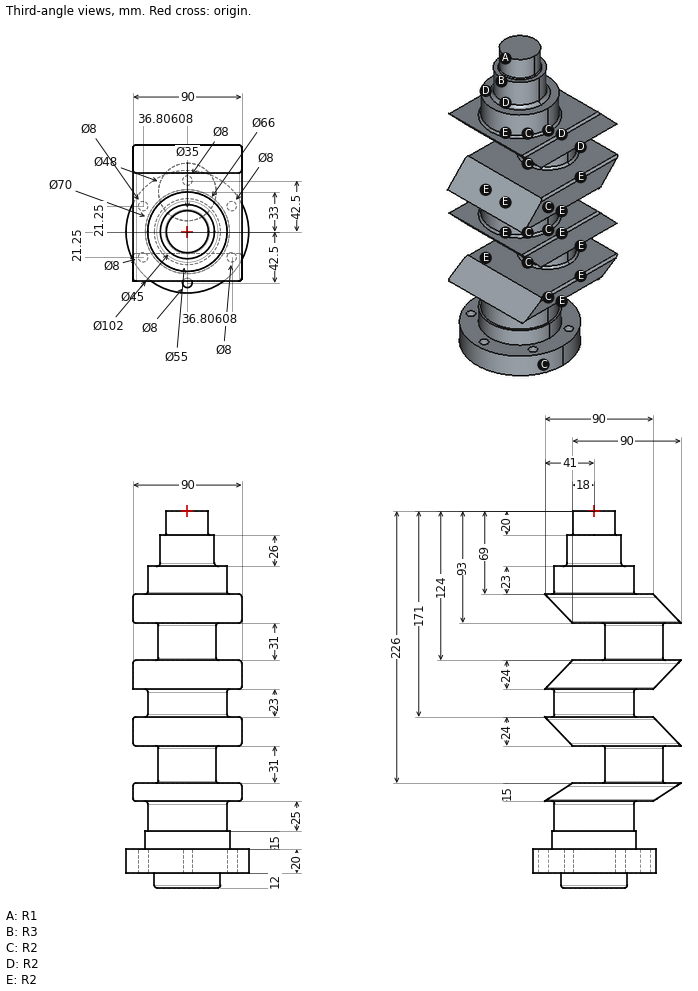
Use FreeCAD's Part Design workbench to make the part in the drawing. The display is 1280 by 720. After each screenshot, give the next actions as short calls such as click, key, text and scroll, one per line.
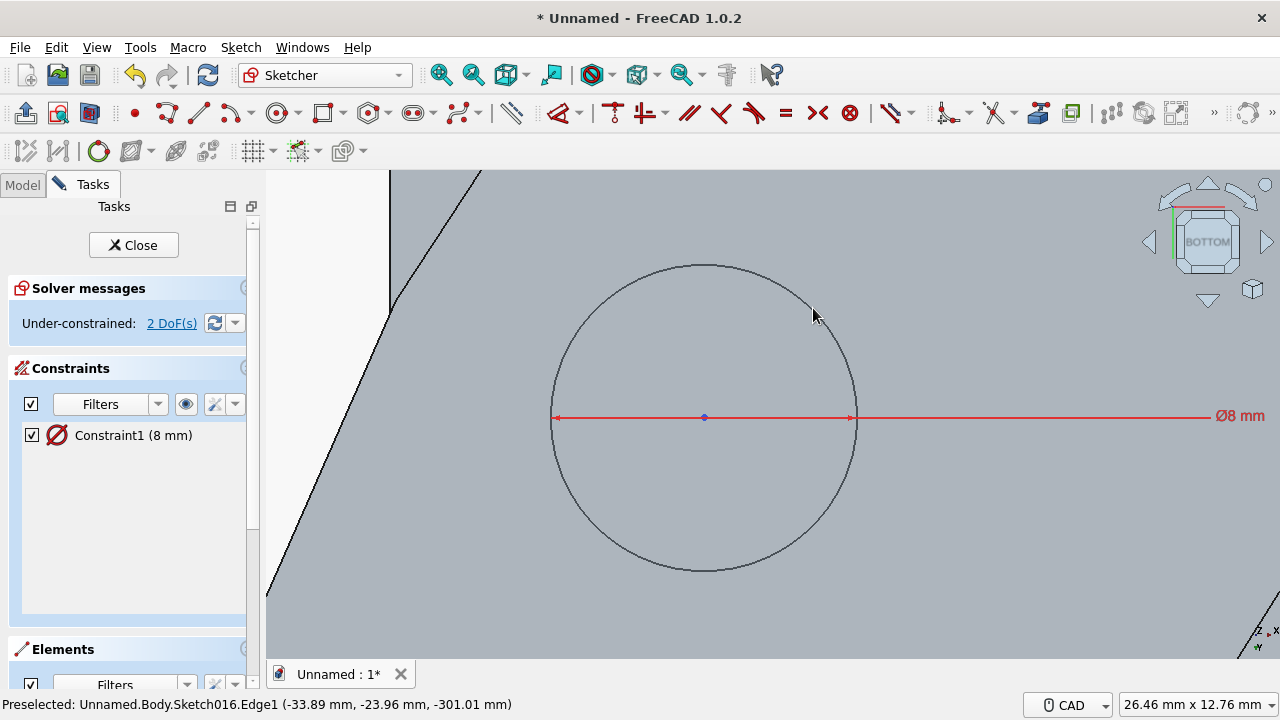
click(558, 114)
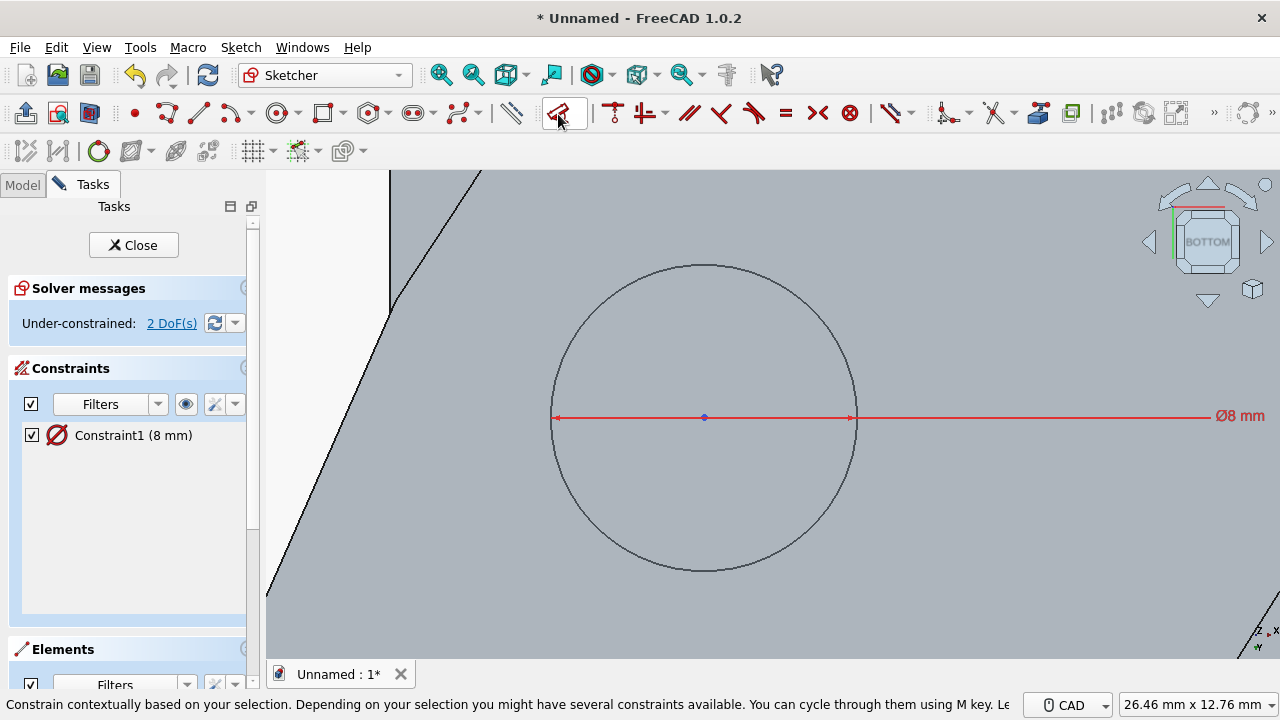
click(704, 418)
click(670, 525)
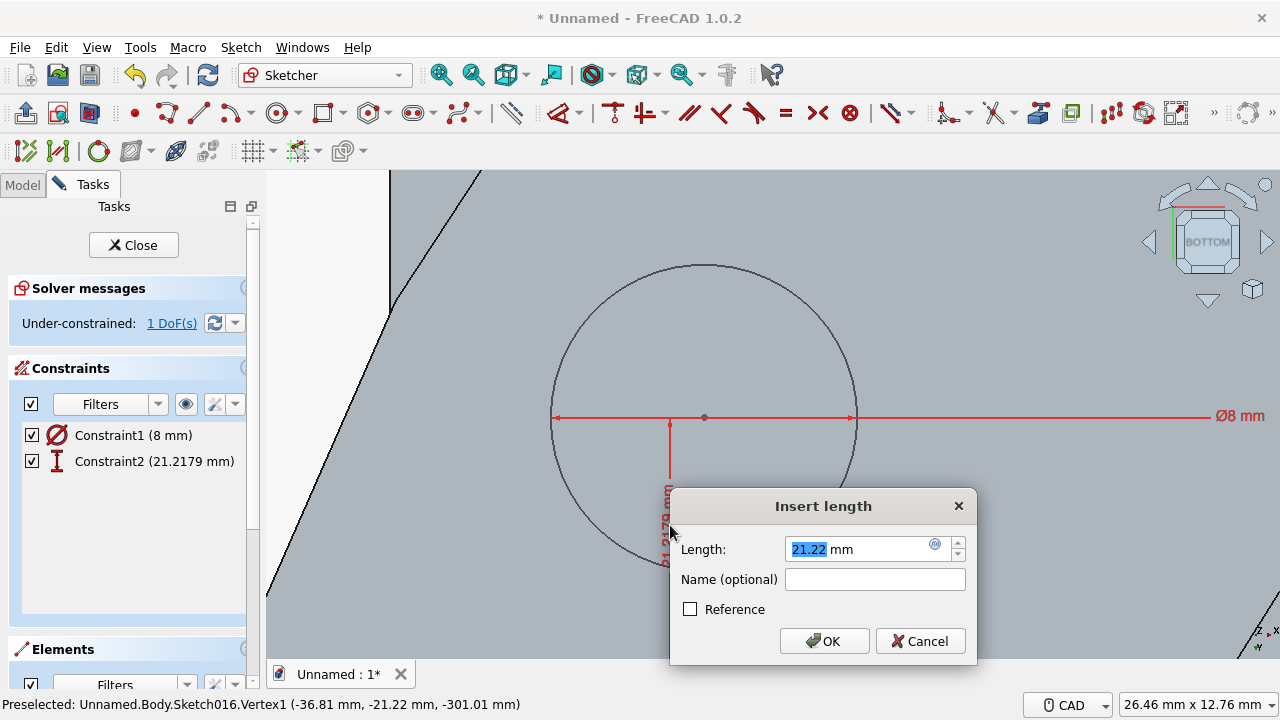
text(21.25)
key(Return)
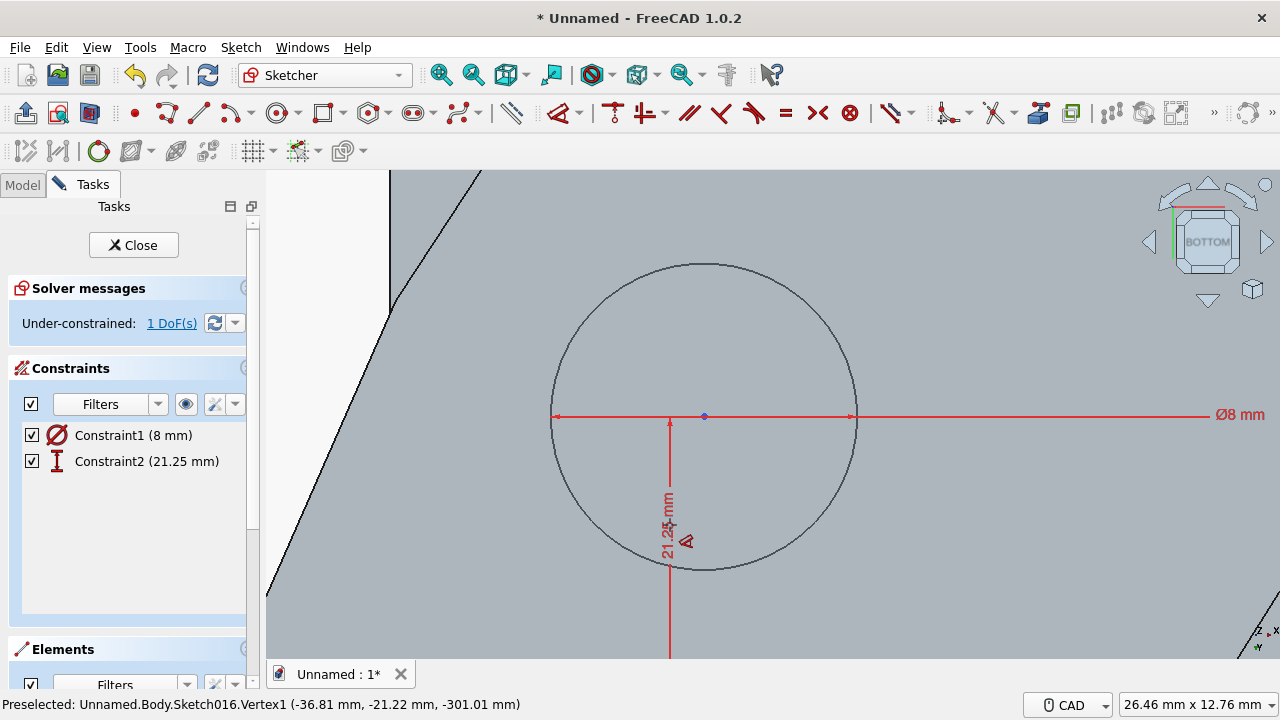
click(704, 417)
click(909, 383)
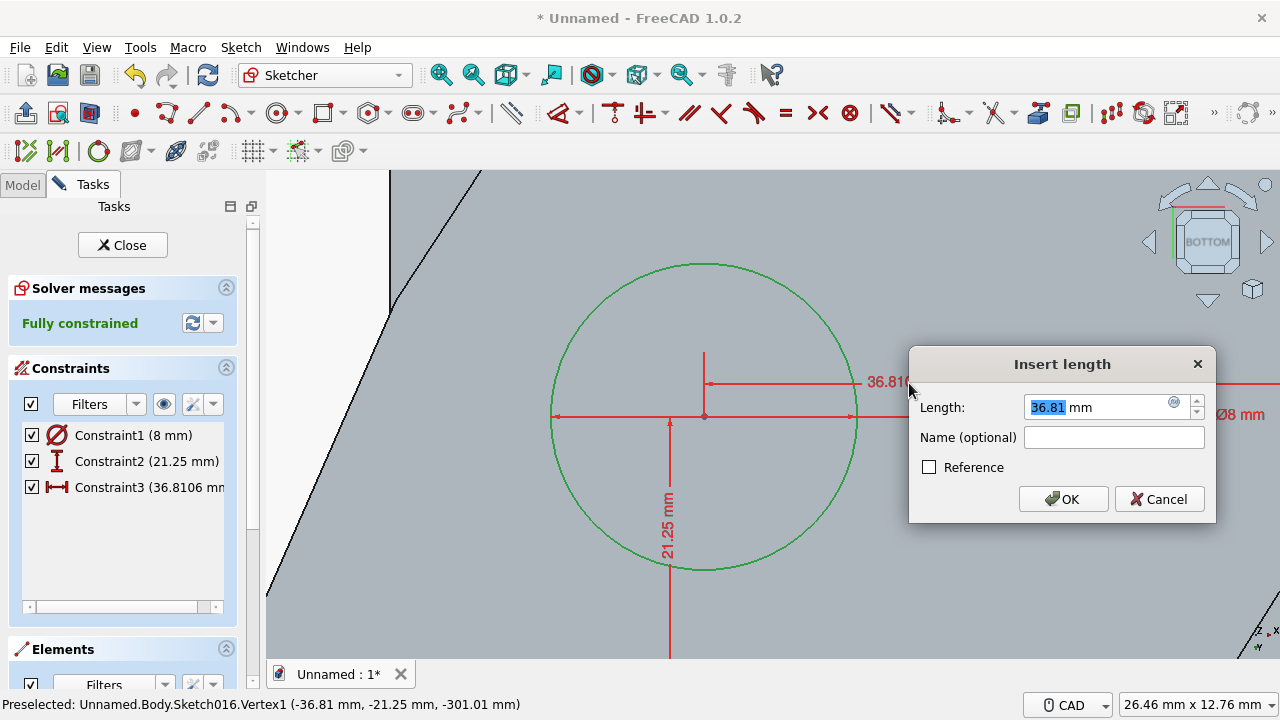
text(36.80608)
key(Return)
key(Escape)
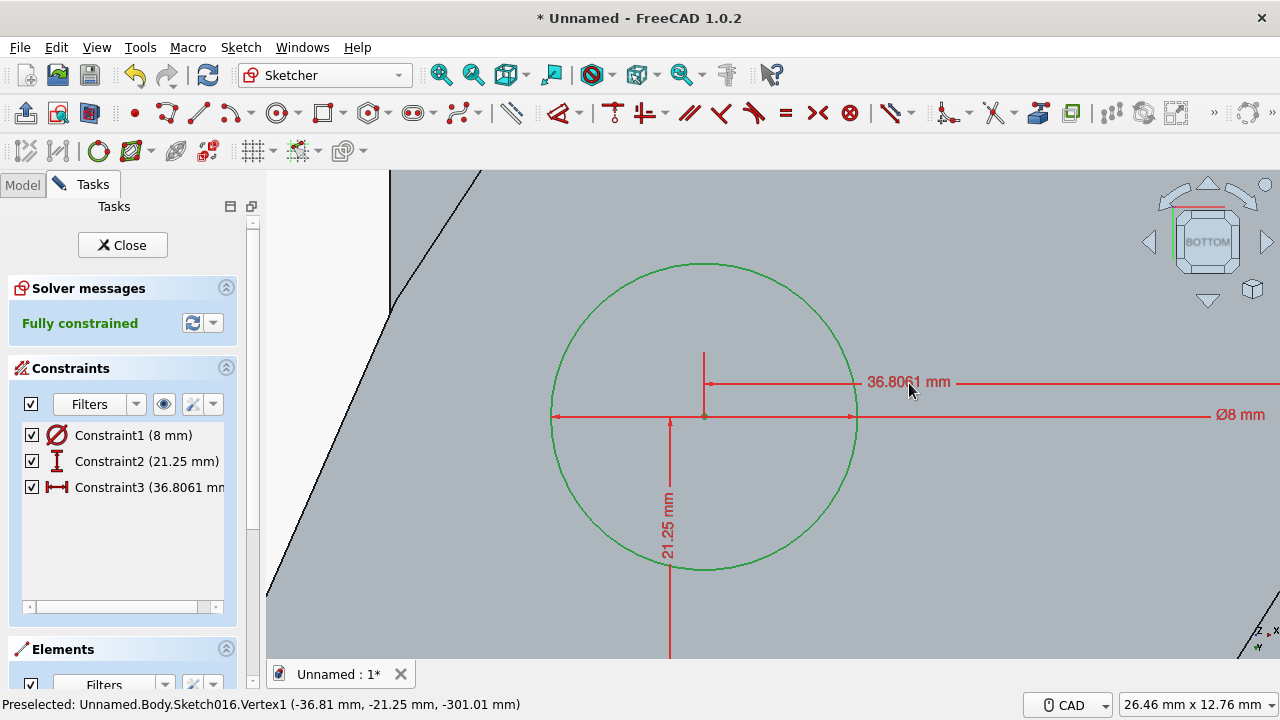
click(123, 245)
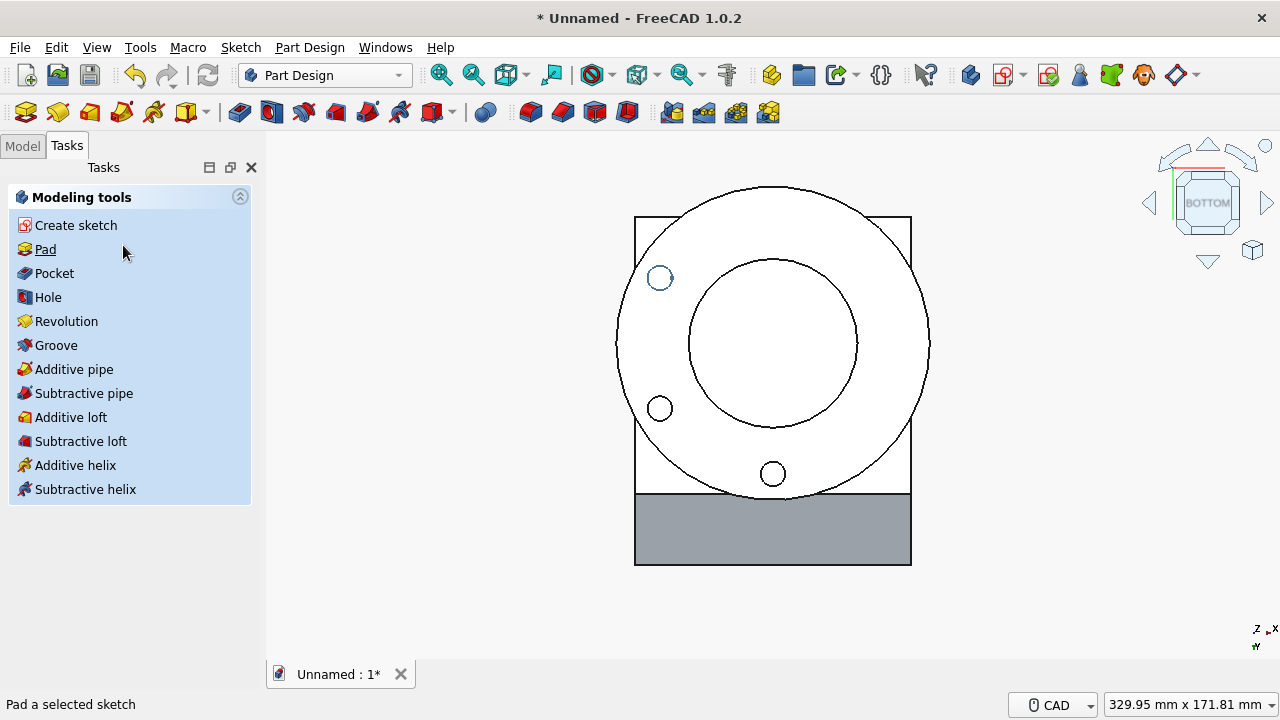
click(240, 112)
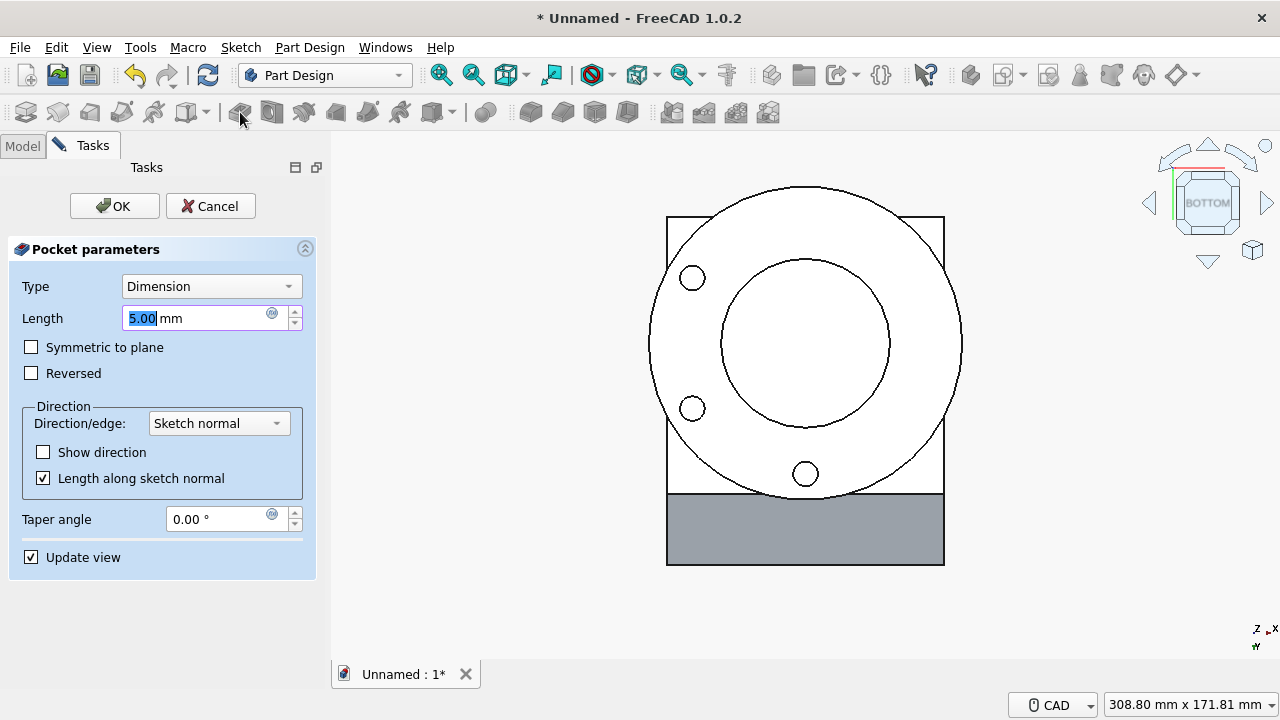
click(212, 286)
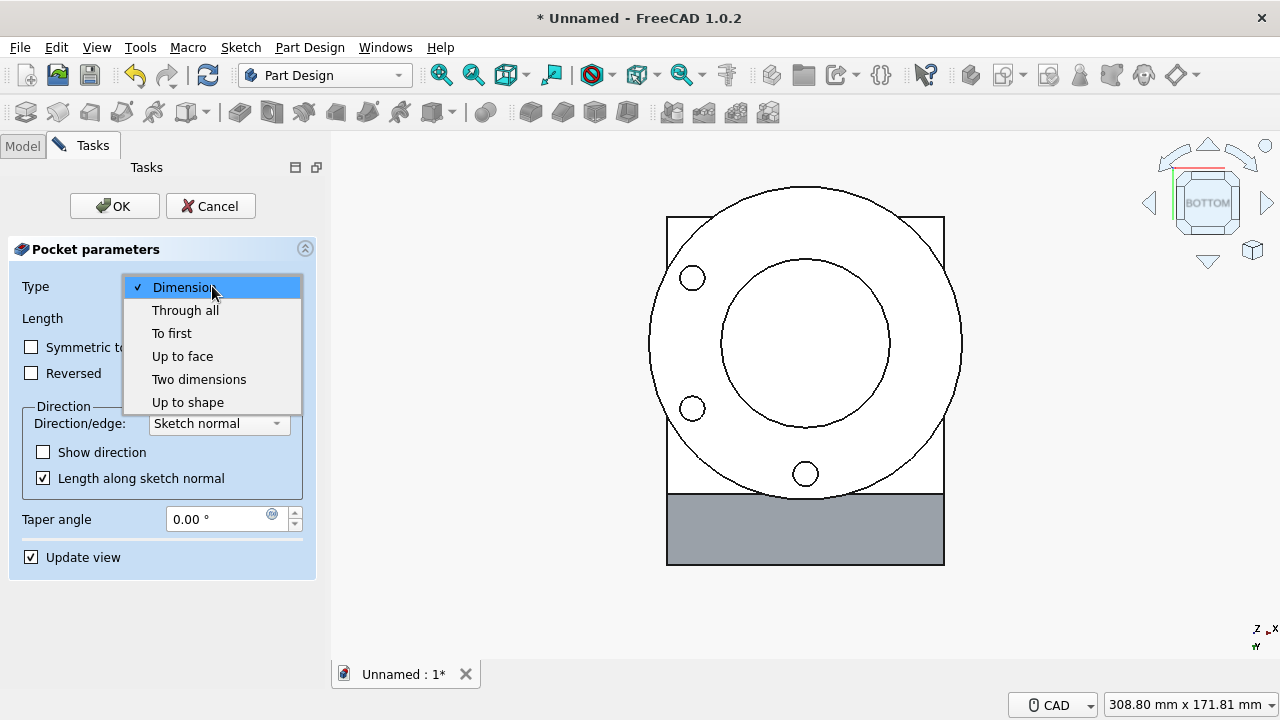
click(212, 334)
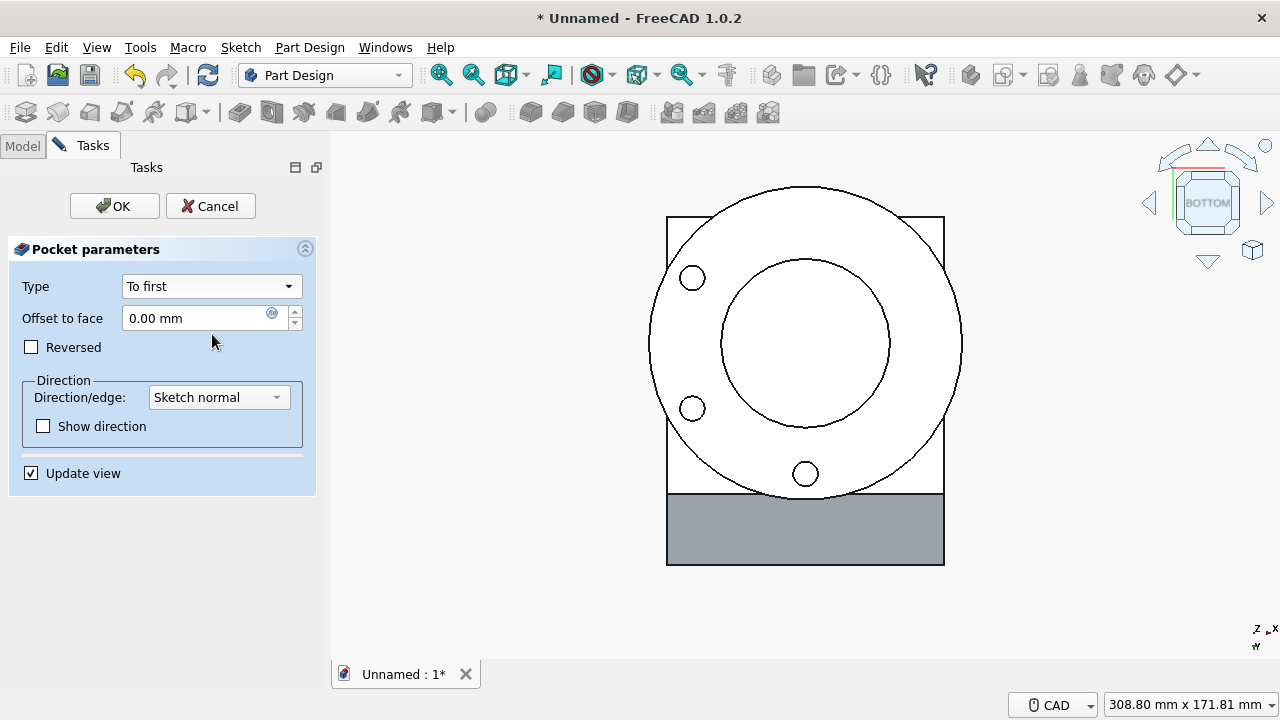
click(115, 206)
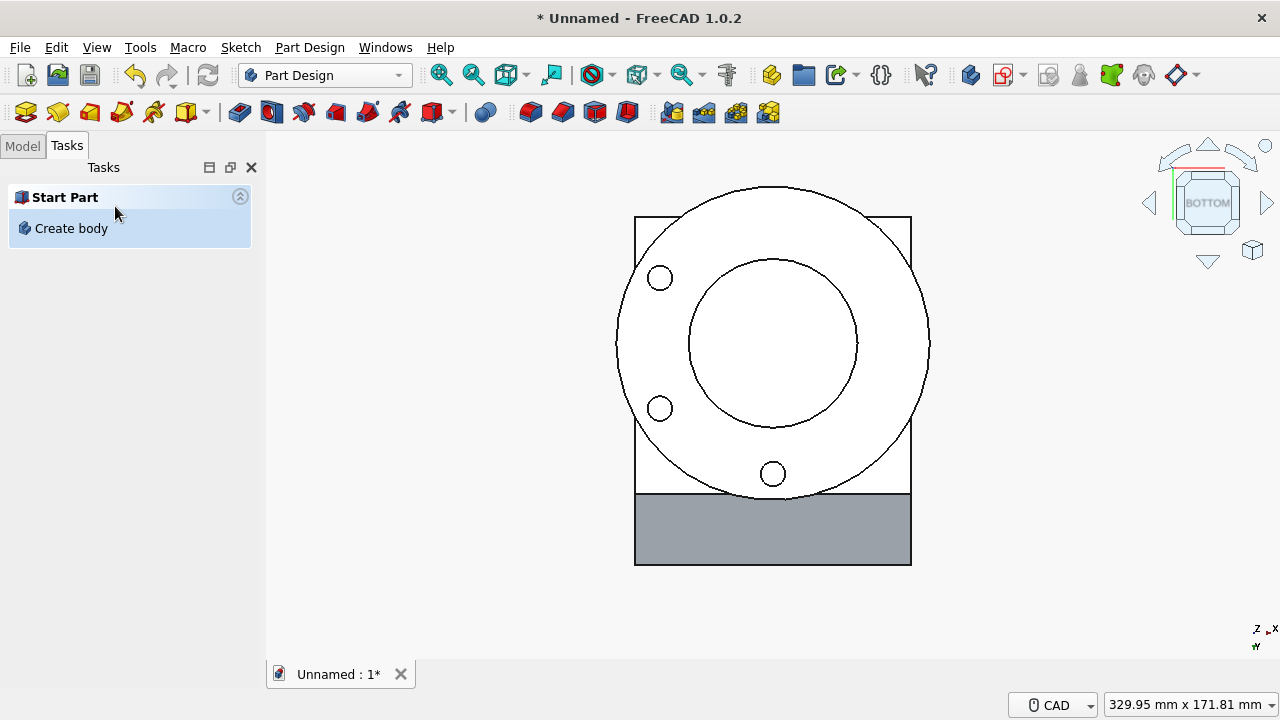
click(863, 432)